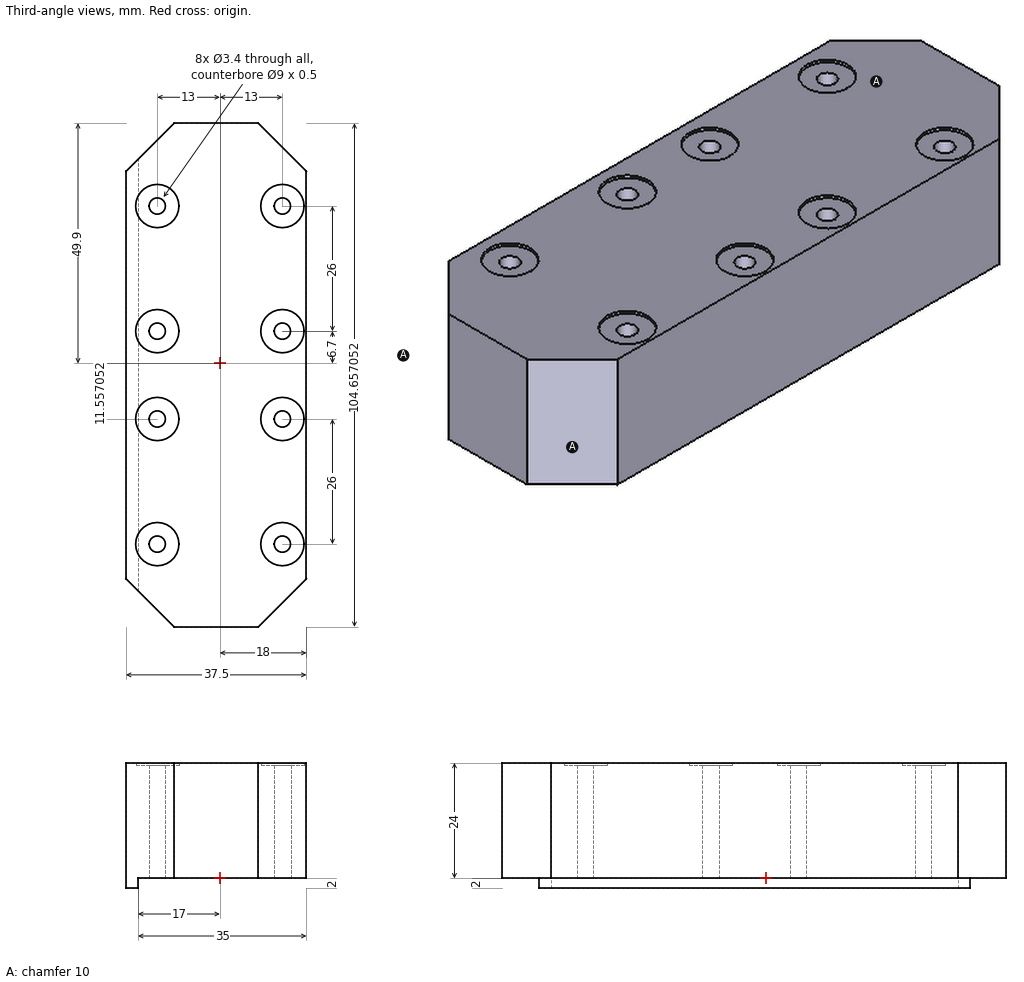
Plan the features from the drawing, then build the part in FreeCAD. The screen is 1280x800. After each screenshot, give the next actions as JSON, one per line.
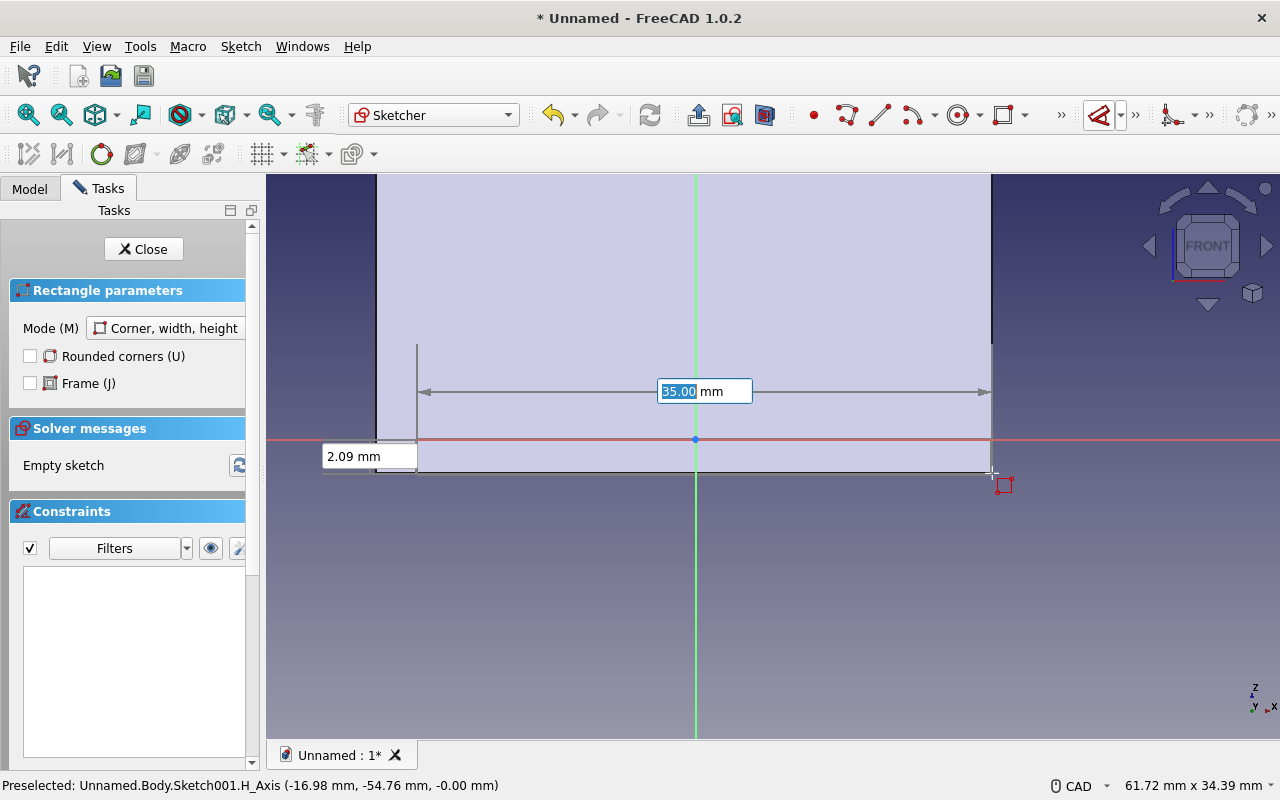
{"action": "type", "text": "35"}
{"action": "key", "text": "Tab"}
{"action": "type", "text": "2"}
{"action": "key", "text": "Return"}
{"action": "key", "text": "Escape"}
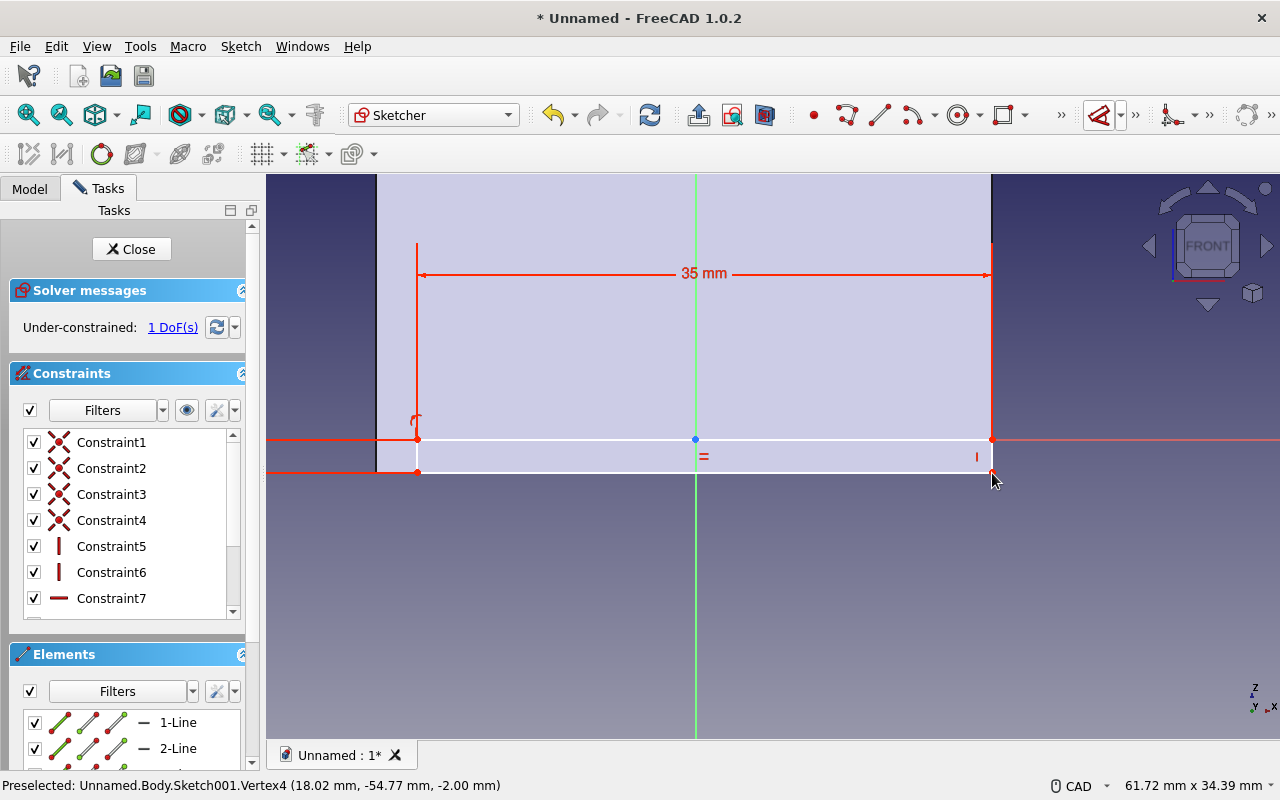
{"action": "left_click", "coordinate": [417, 440]}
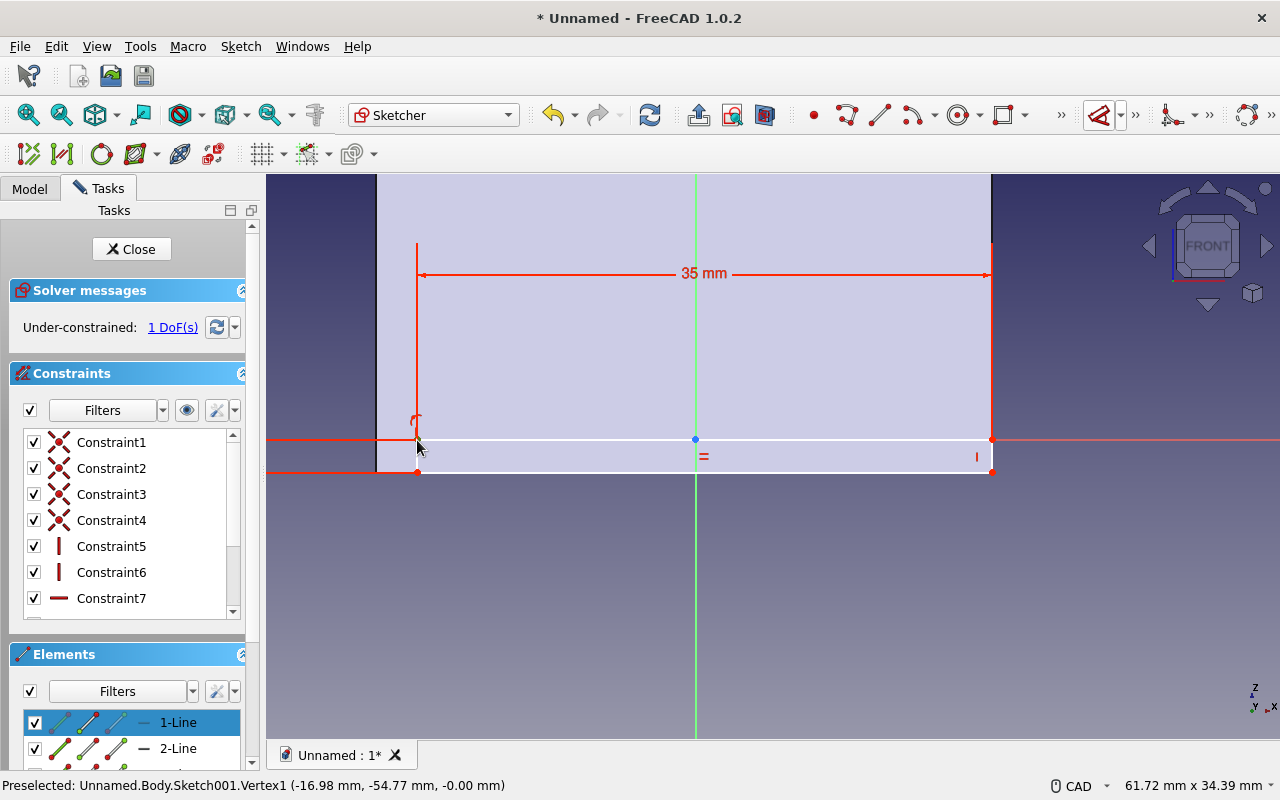
{"action": "key", "text": "l"}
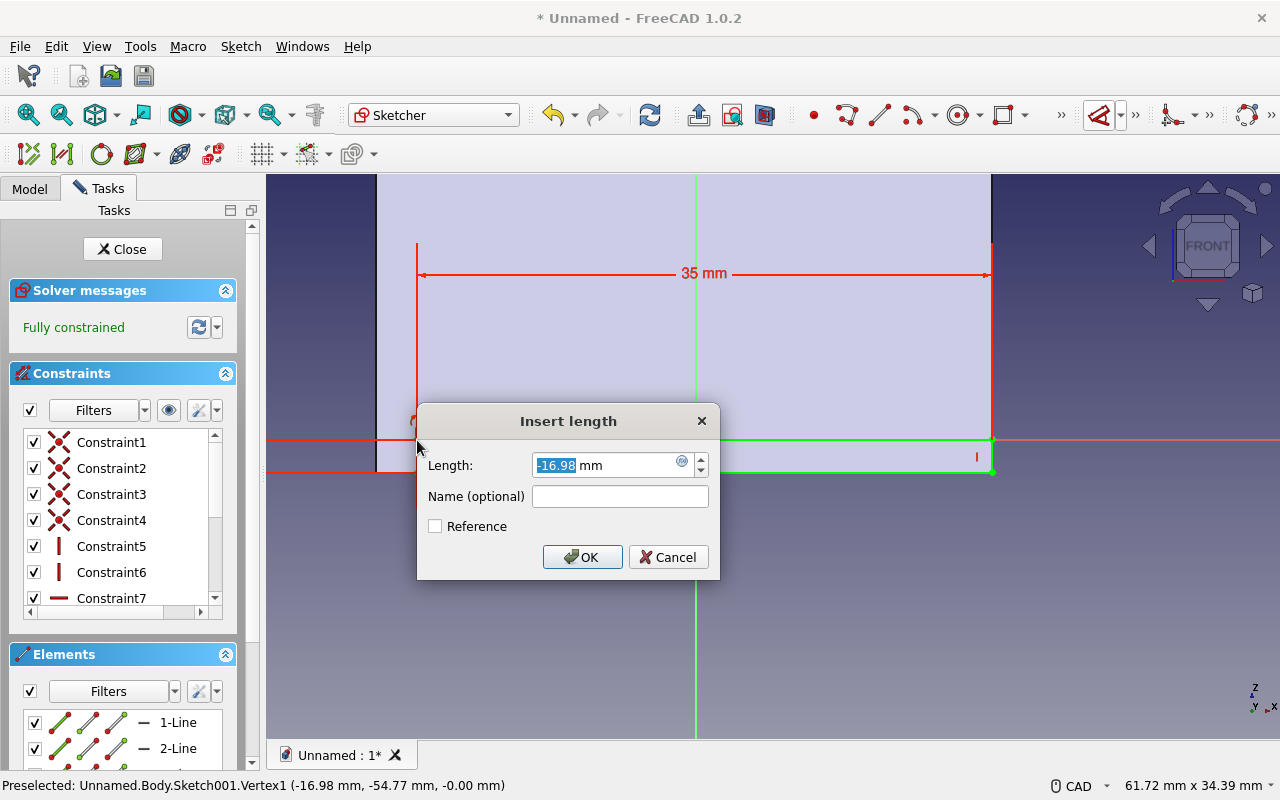
{"action": "type", "text": "-17"}
{"action": "key", "text": "Return"}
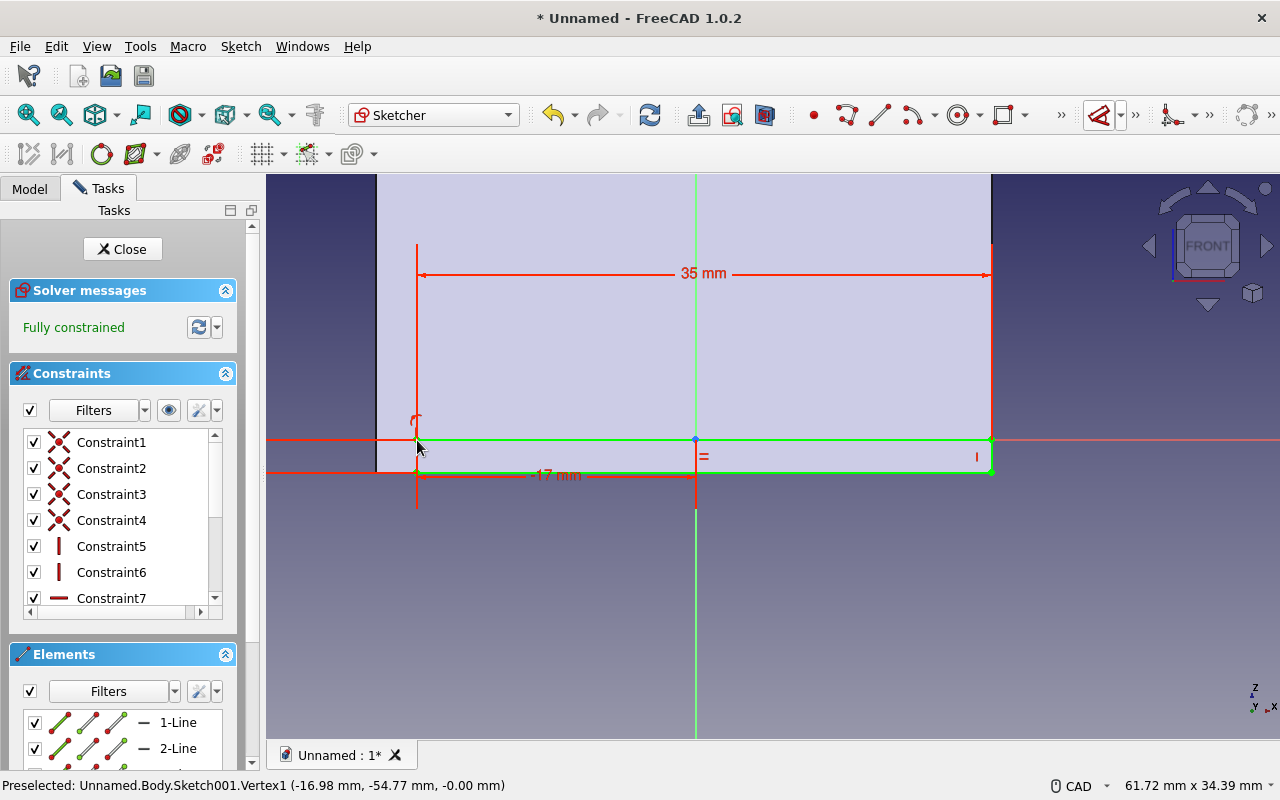
{"action": "left_click", "coordinate": [123, 249]}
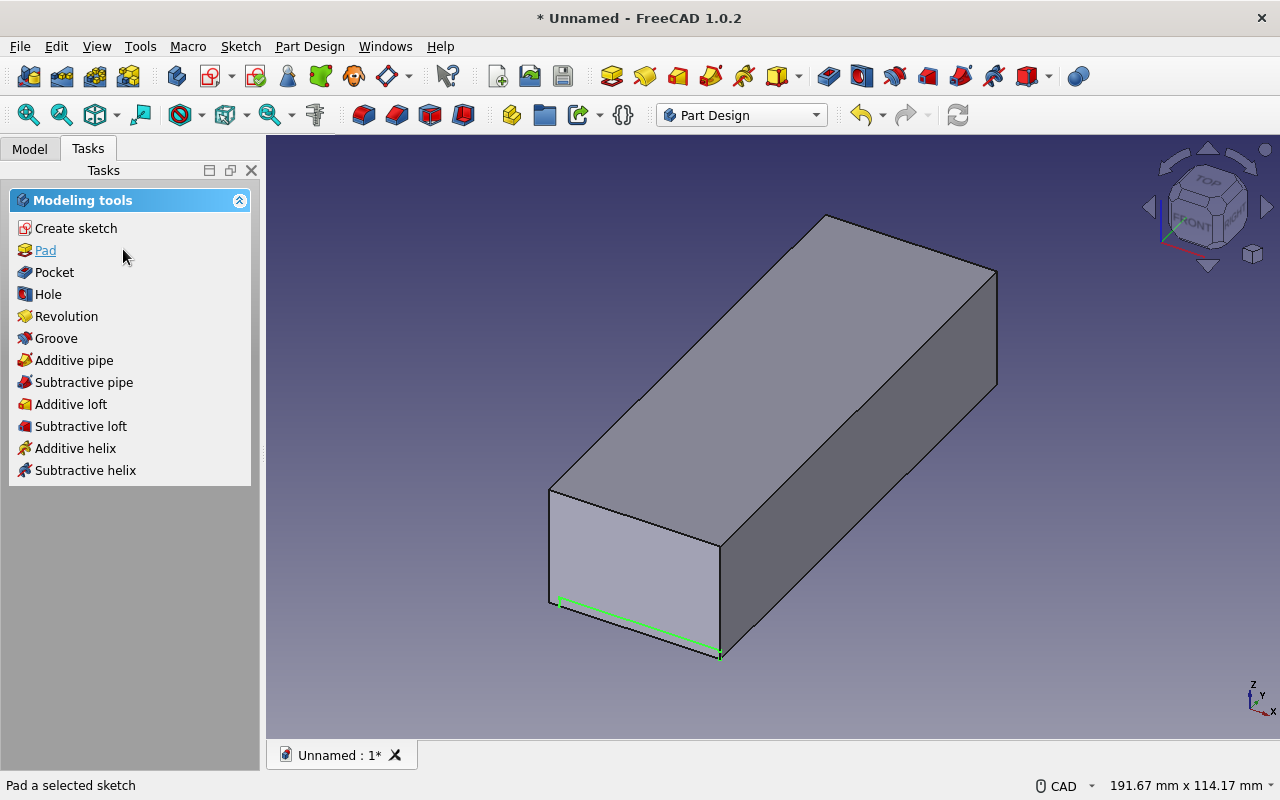
{"action": "left_click", "coordinate": [829, 76]}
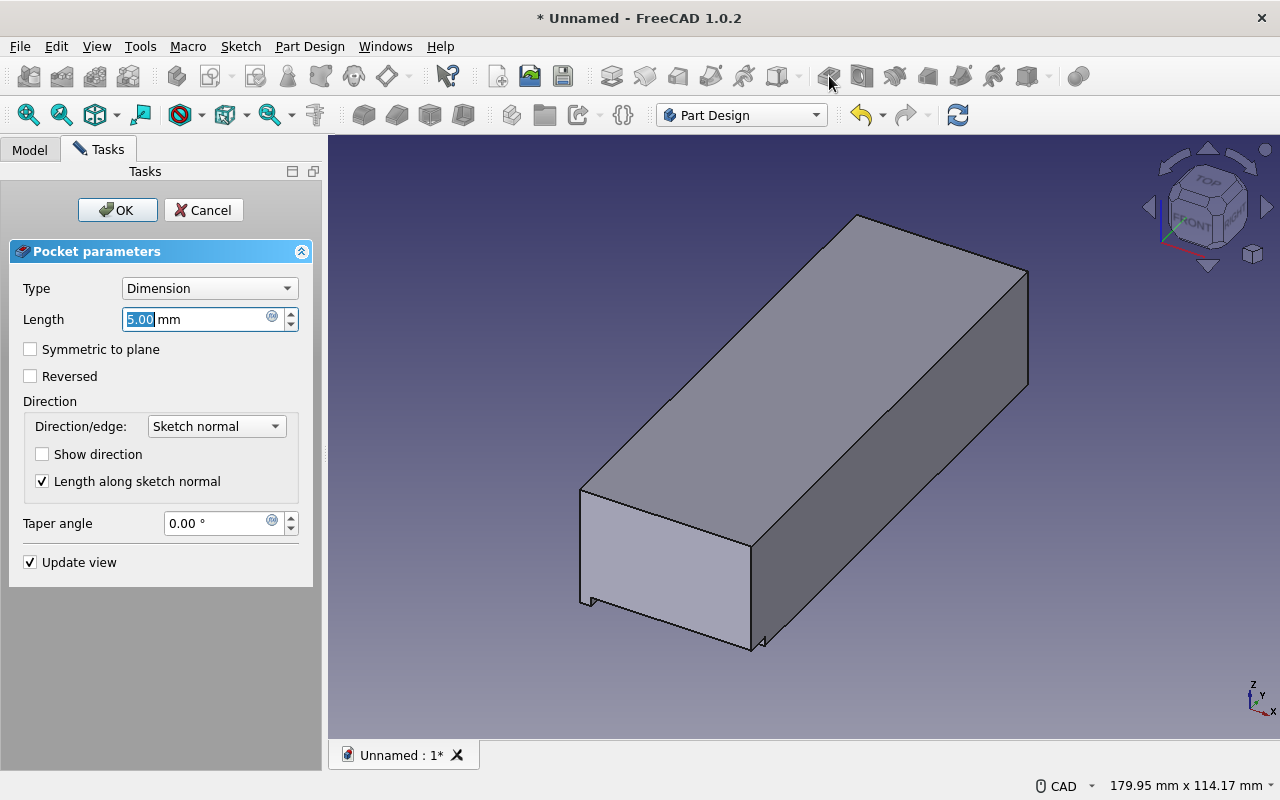
{"action": "left_click", "coordinate": [210, 288]}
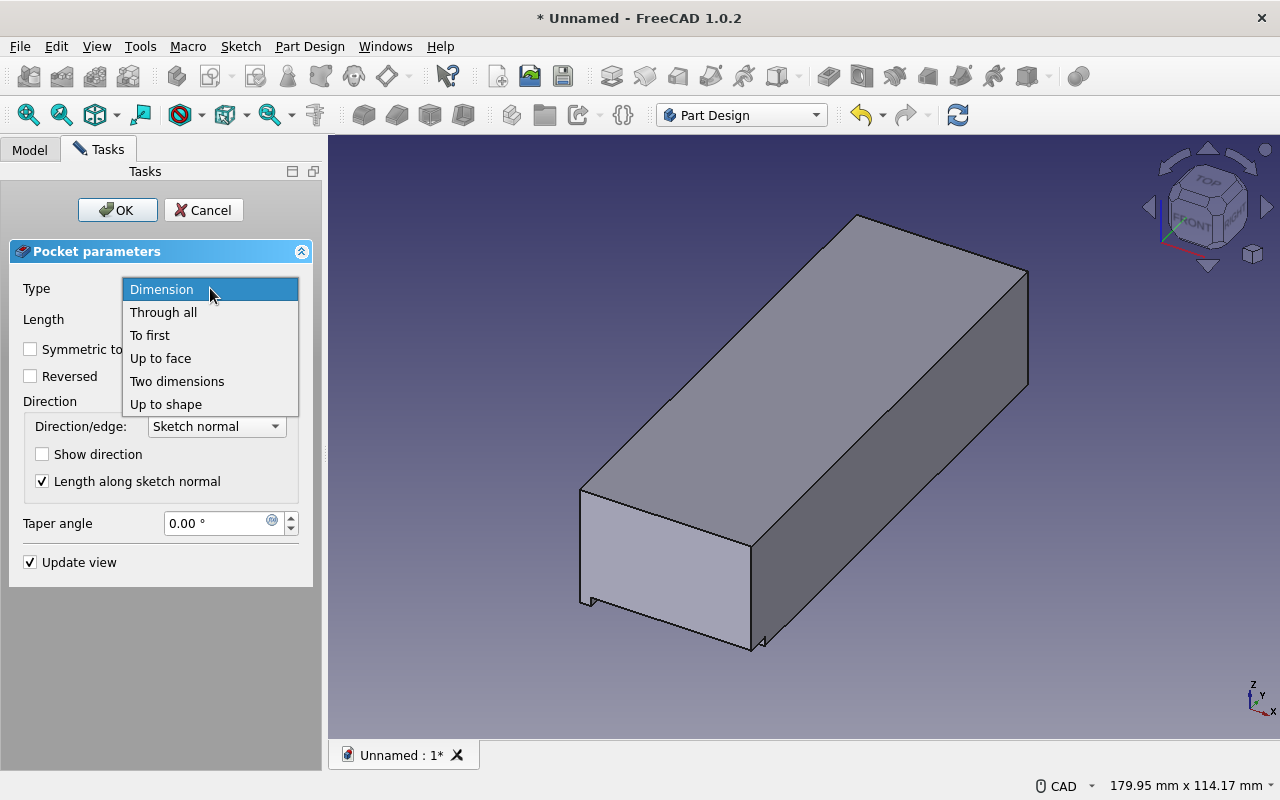
{"action": "left_click", "coordinate": [208, 312]}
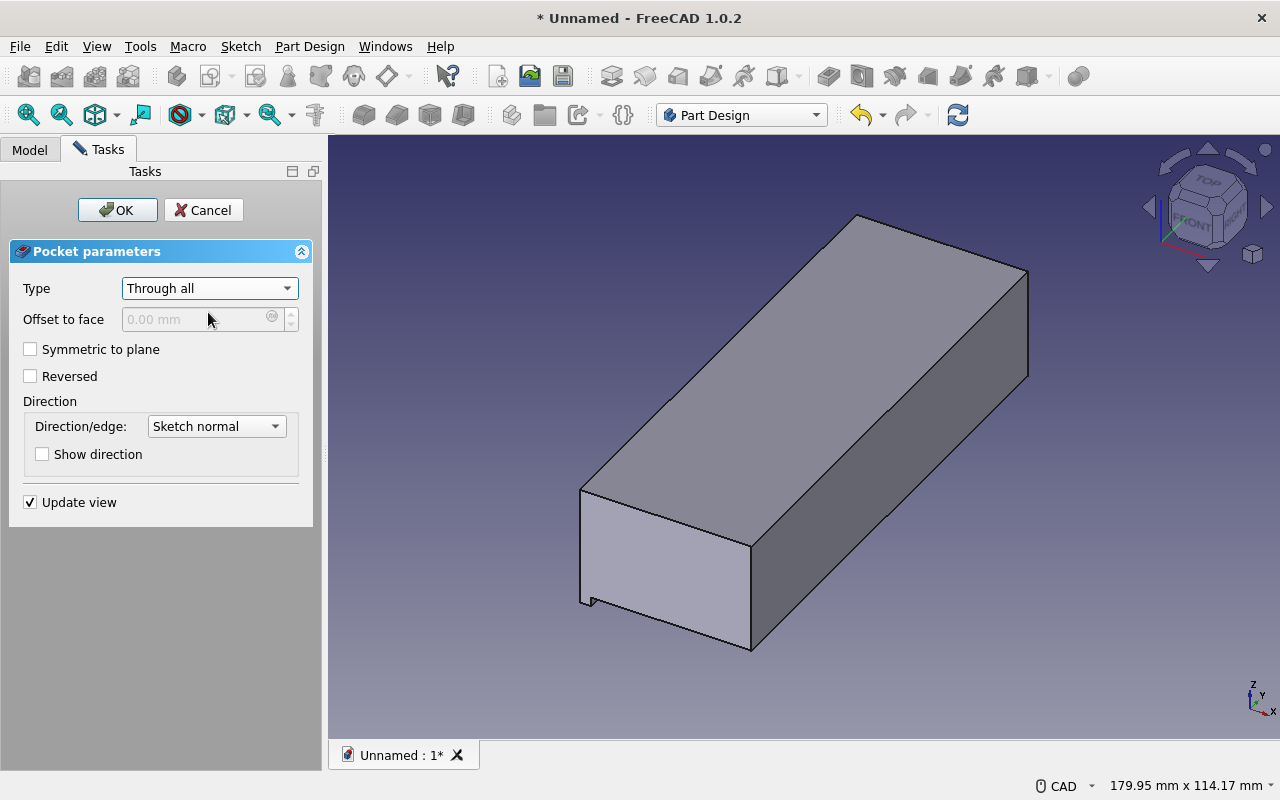
{"action": "left_click", "coordinate": [118, 210]}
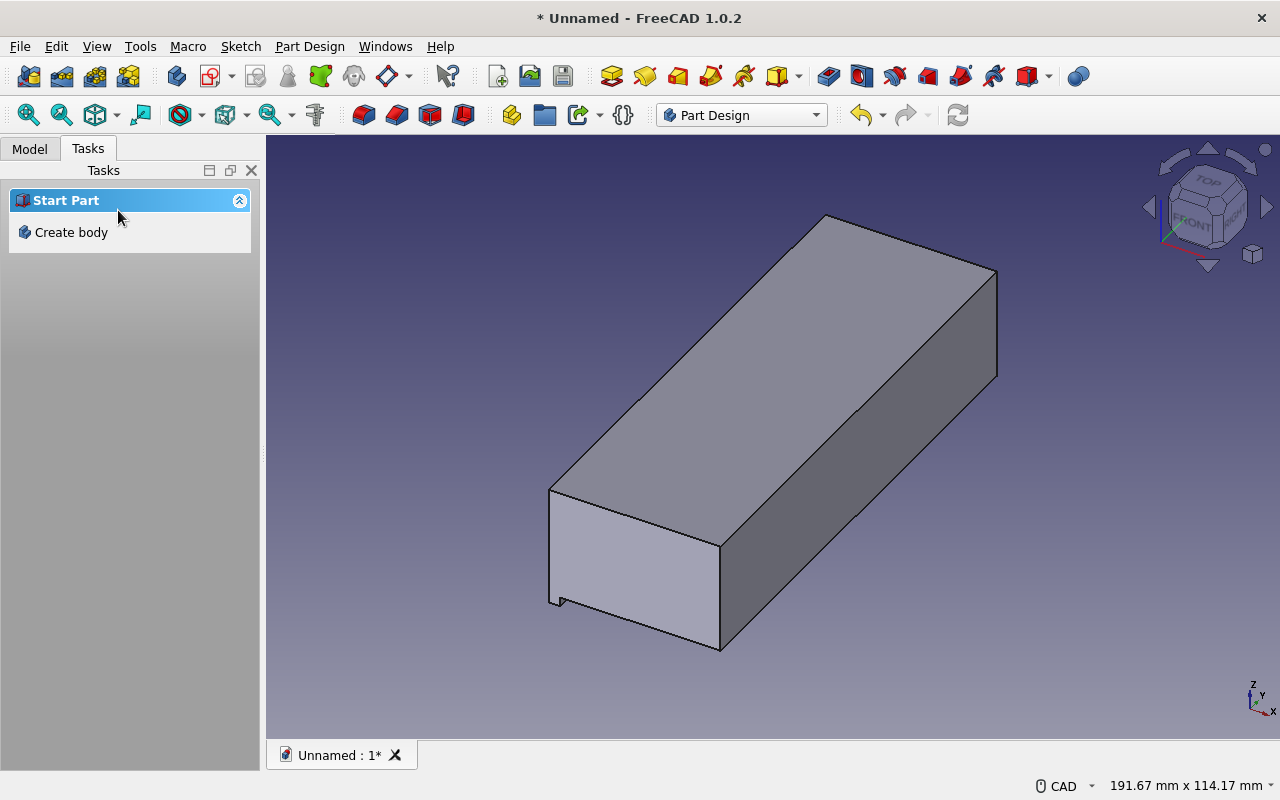
{"action": "left_click", "coordinate": [720, 598]}